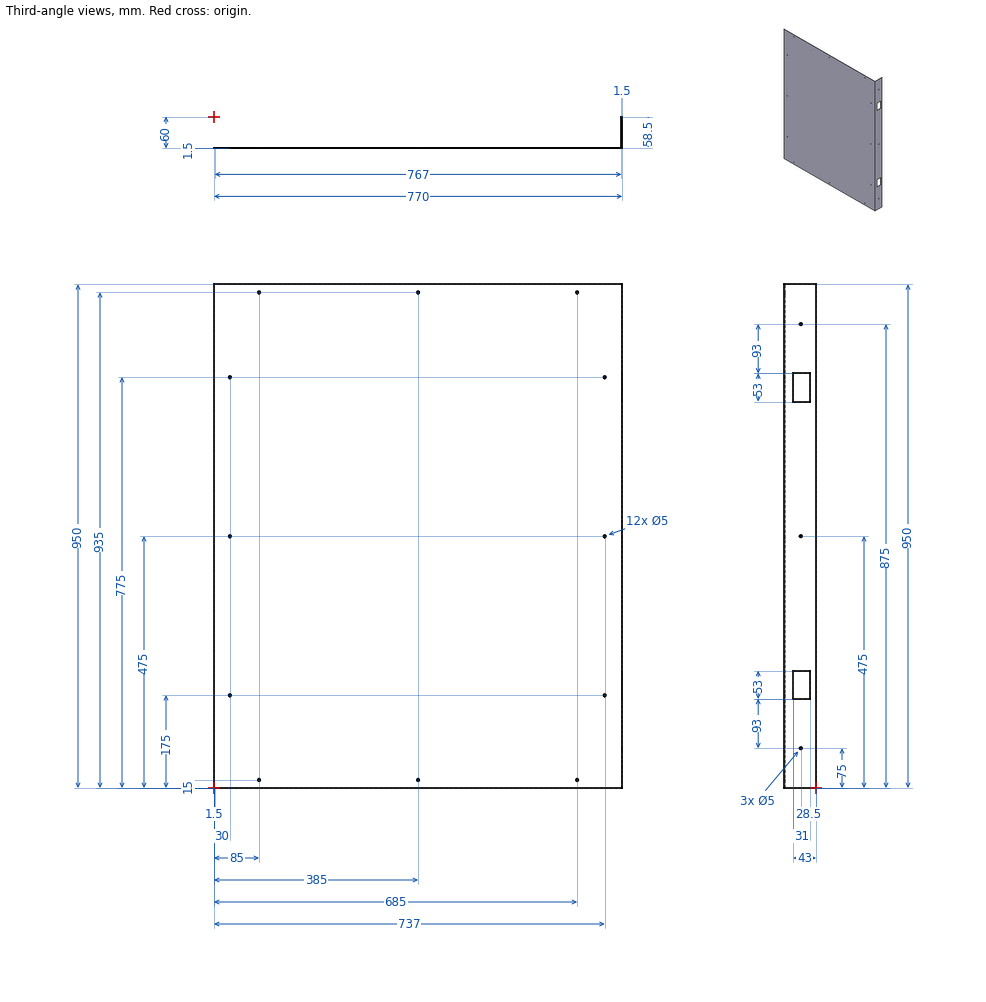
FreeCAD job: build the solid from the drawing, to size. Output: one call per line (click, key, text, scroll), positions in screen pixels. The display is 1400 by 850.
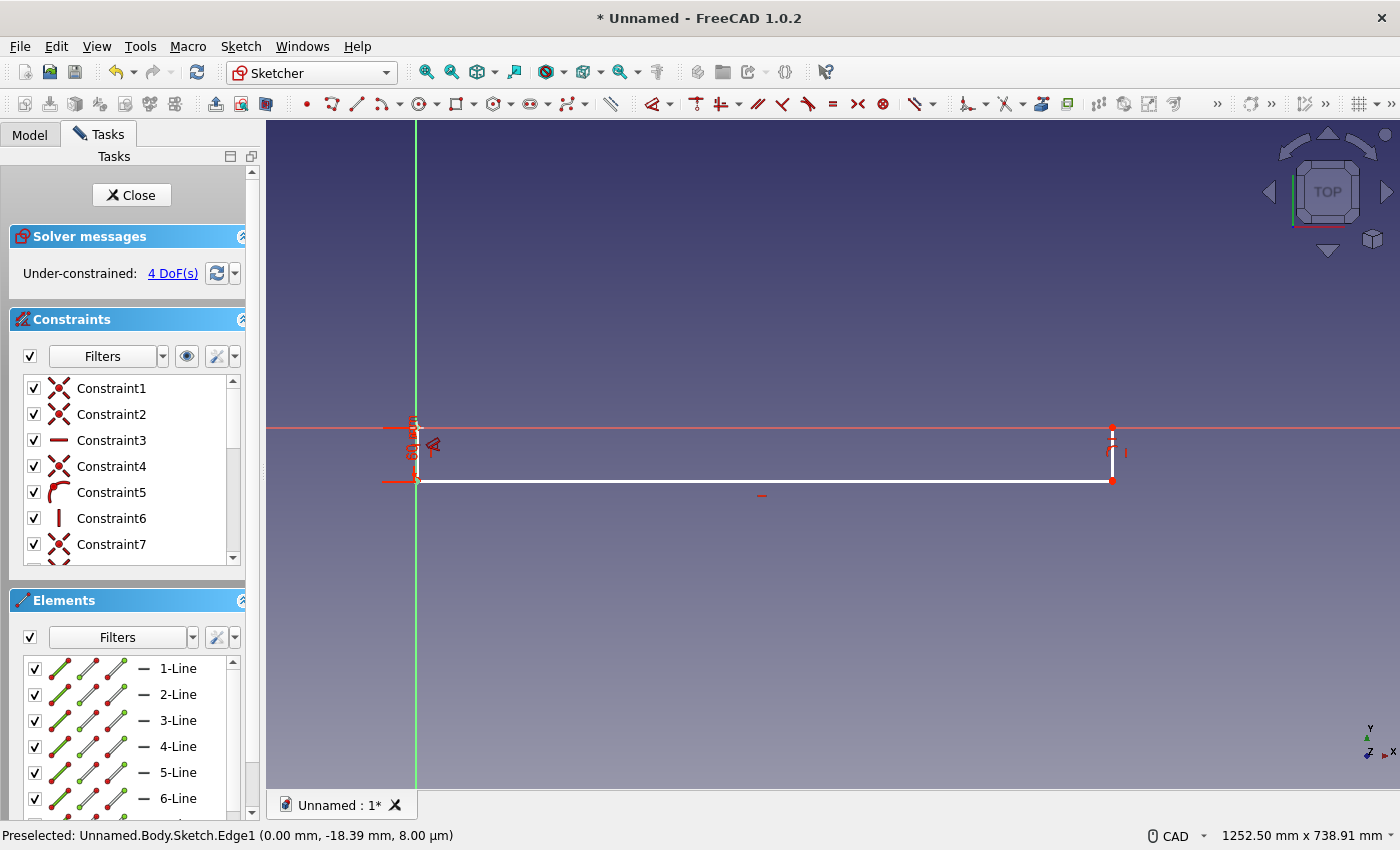
scroll(625, 482, up, 12)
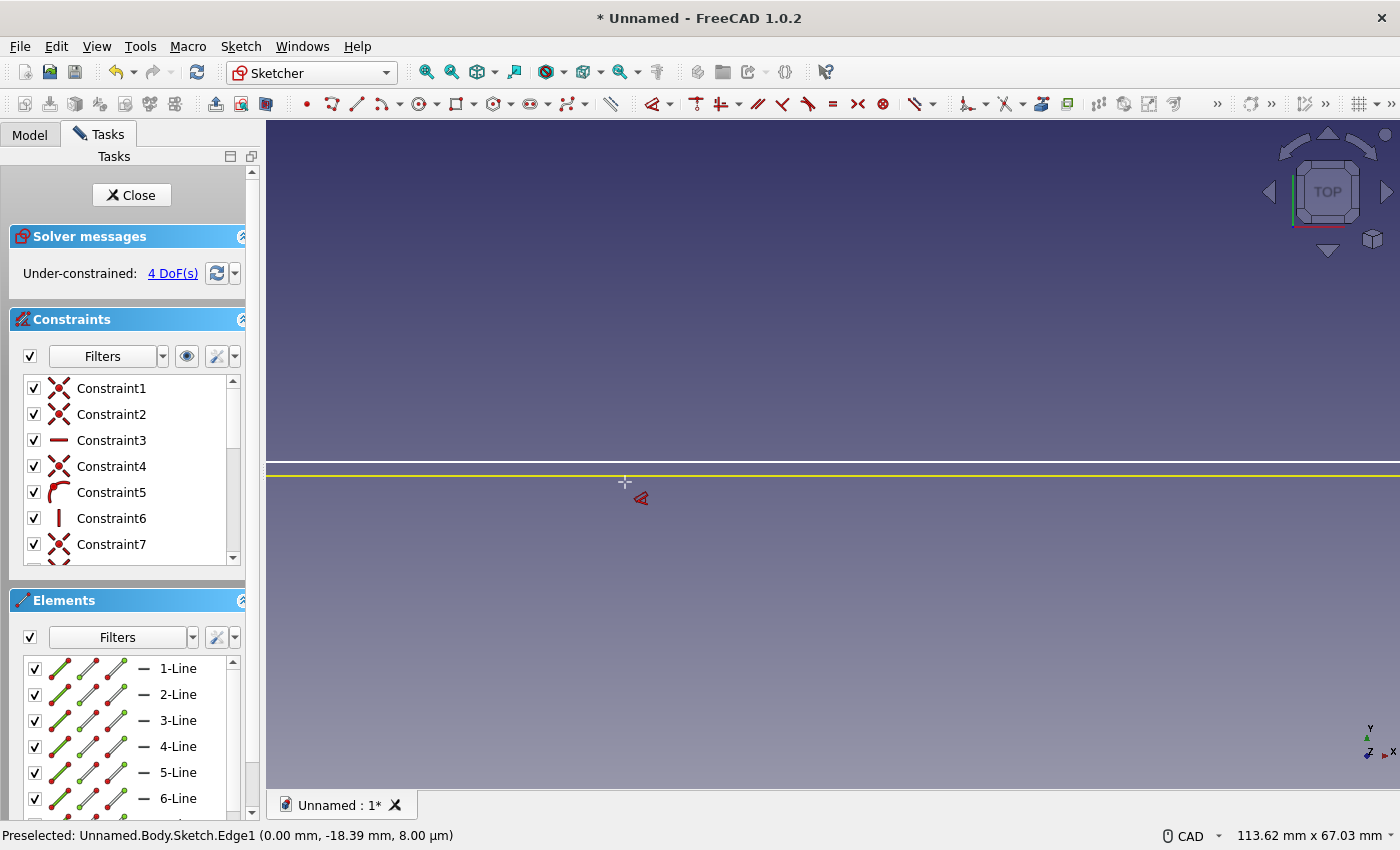
click(625, 476)
click(764, 510)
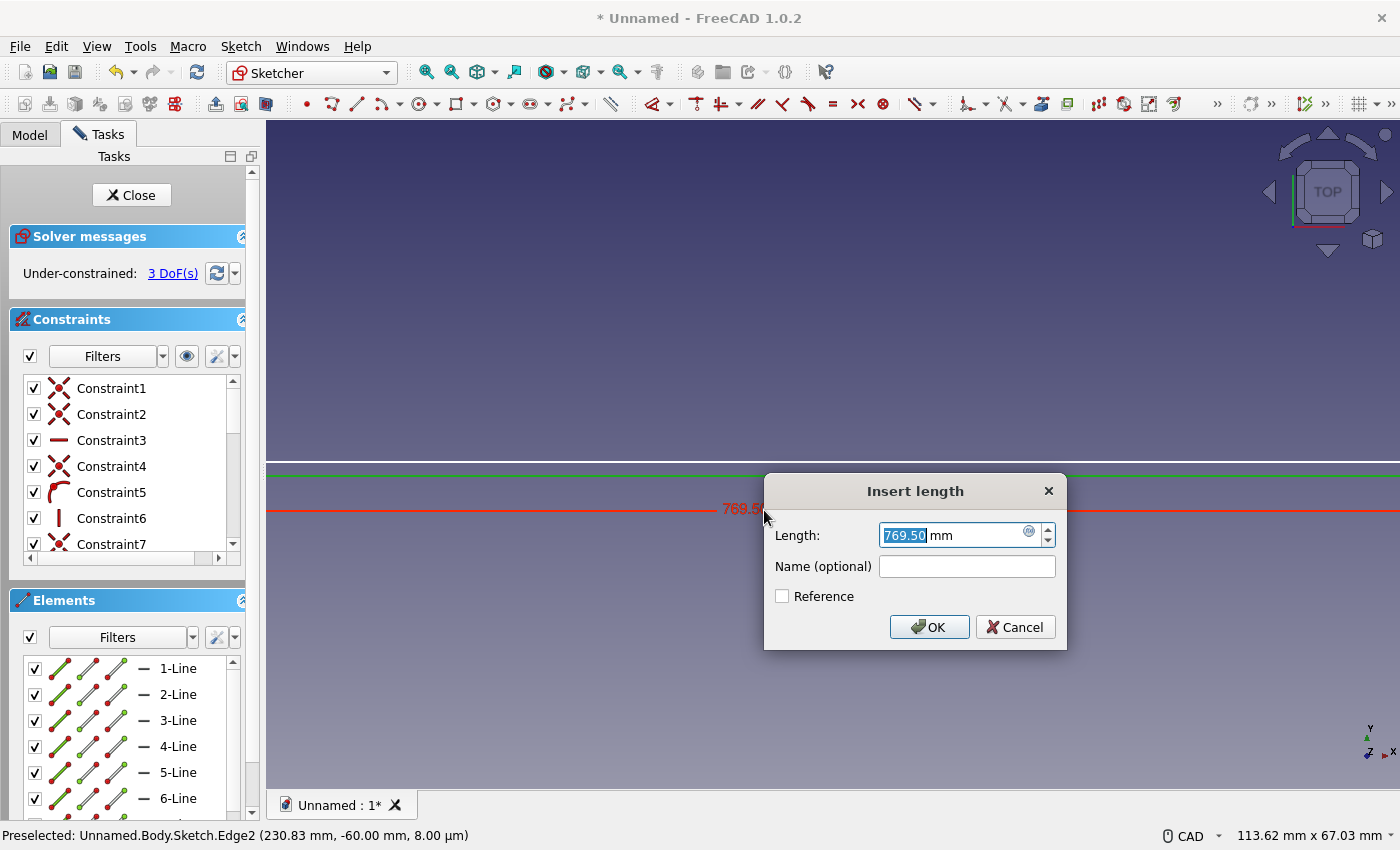
text(770)
key(Return)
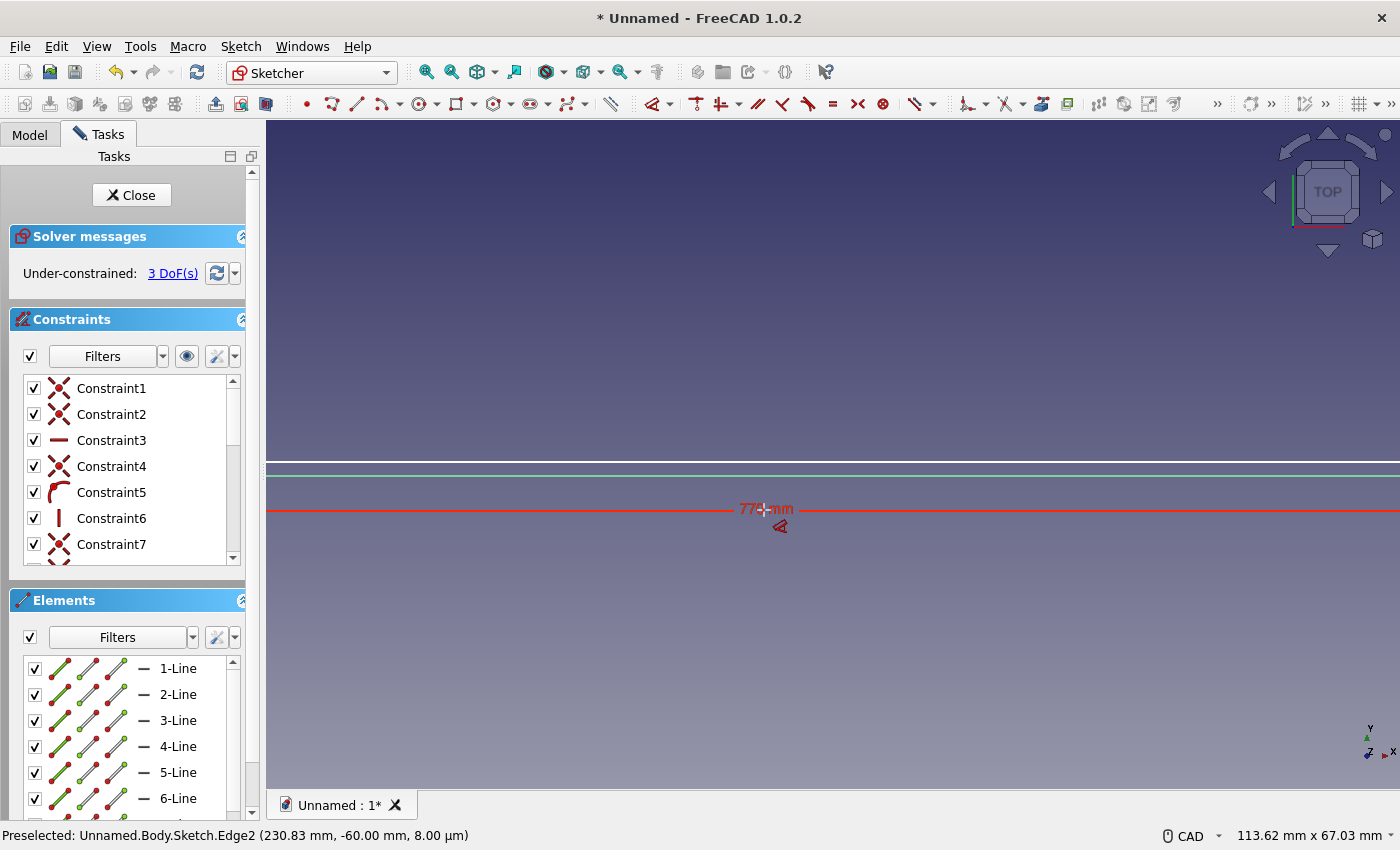
scroll(625, 482, down, 12)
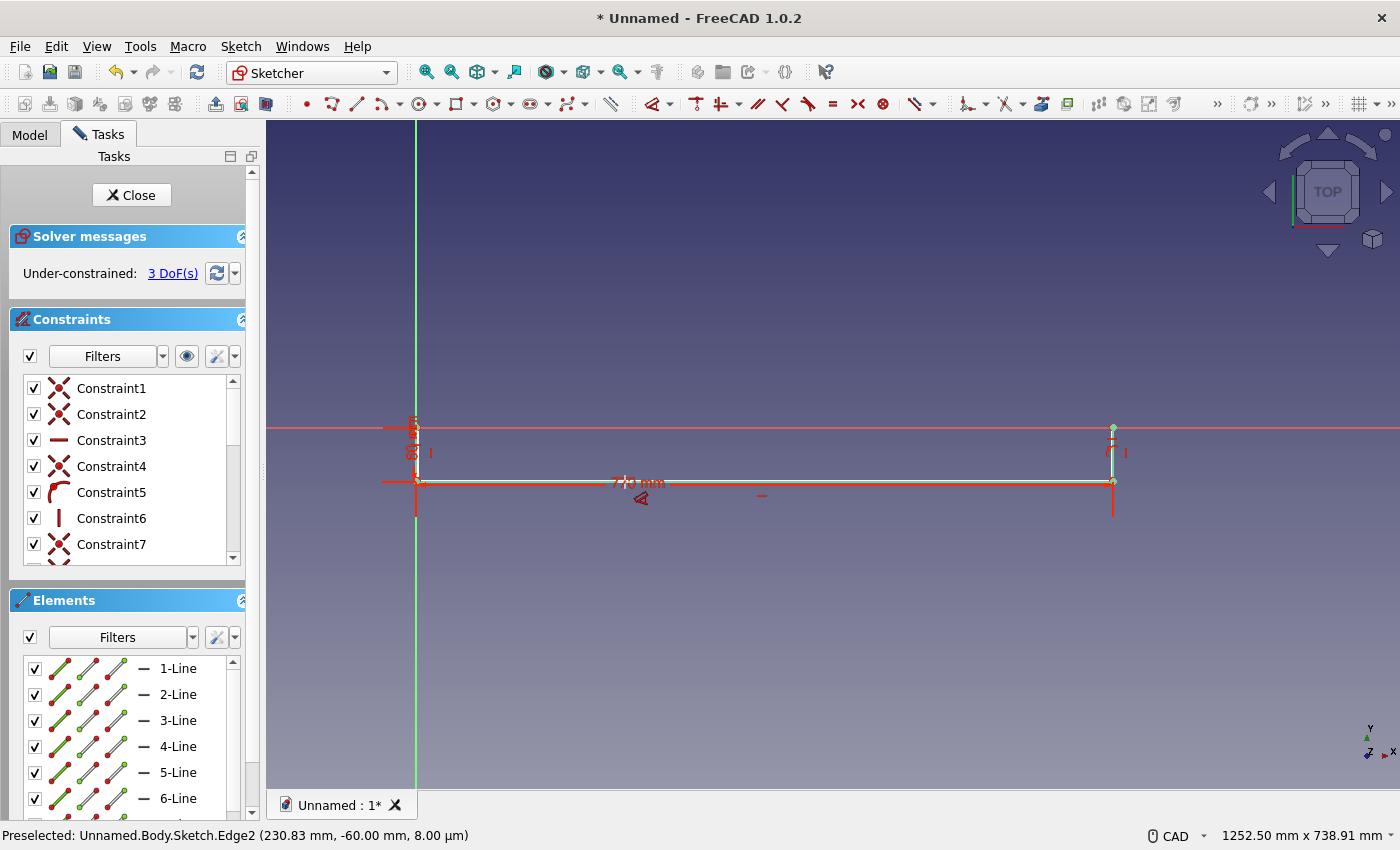
scroll(1113, 428, up, 17)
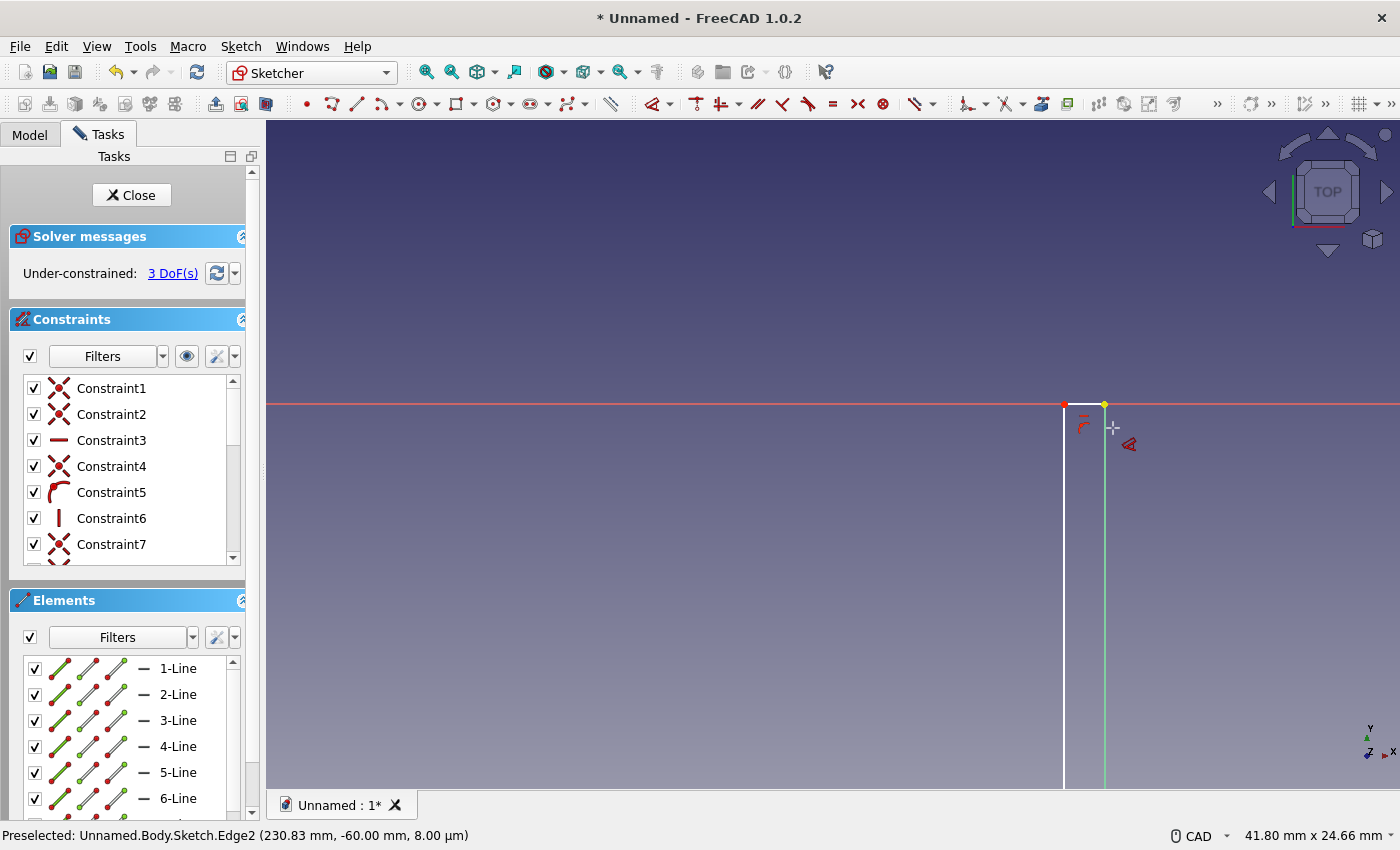
click(1085, 404)
click(1085, 370)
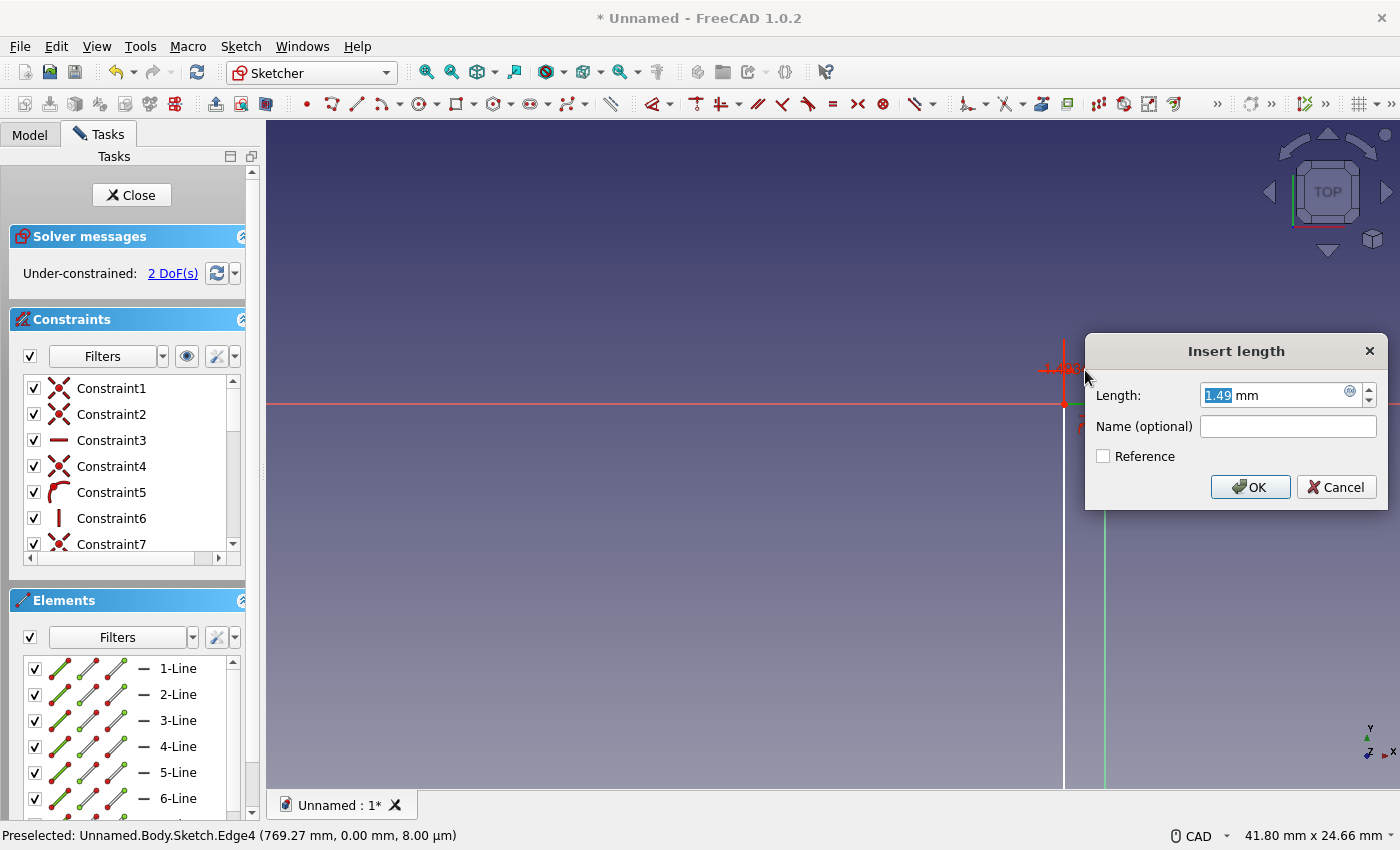
text(1.5)
key(Return)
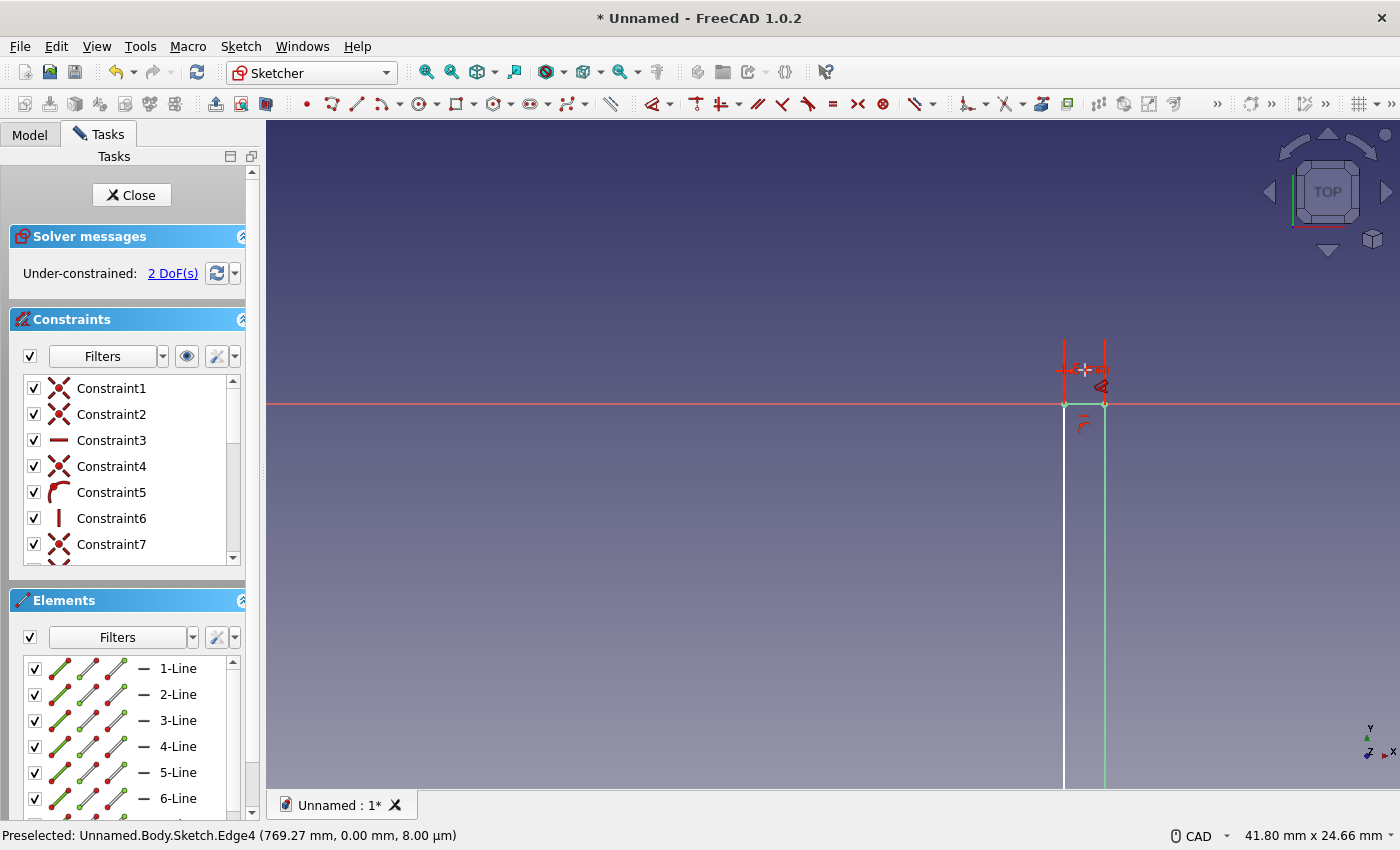
scroll(1194, 422, down, 16)